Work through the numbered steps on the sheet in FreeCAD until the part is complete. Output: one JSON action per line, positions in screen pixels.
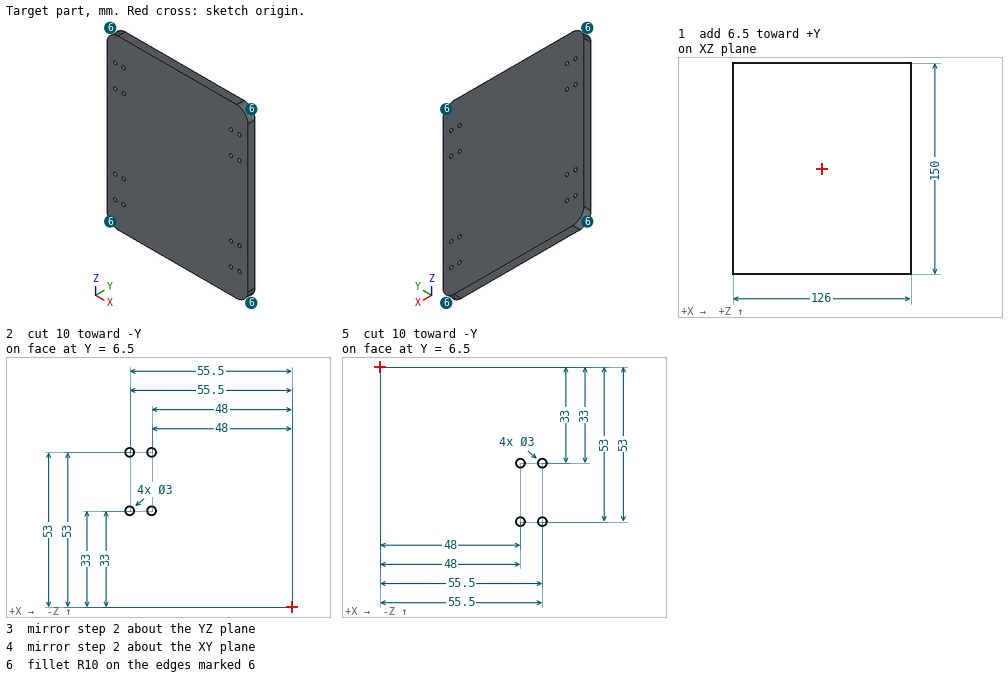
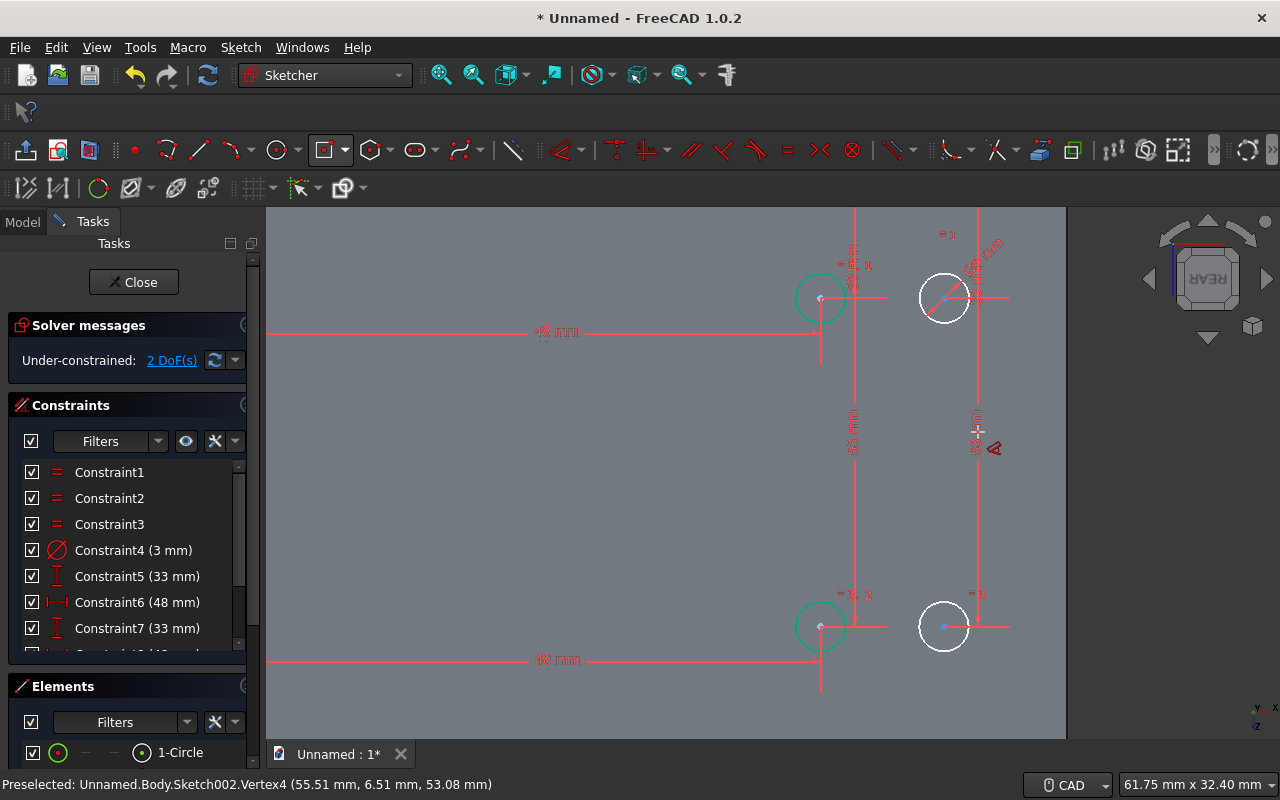
{"action": "left_click", "coordinate": [944, 298]}
{"action": "left_click", "coordinate": [470, 332]}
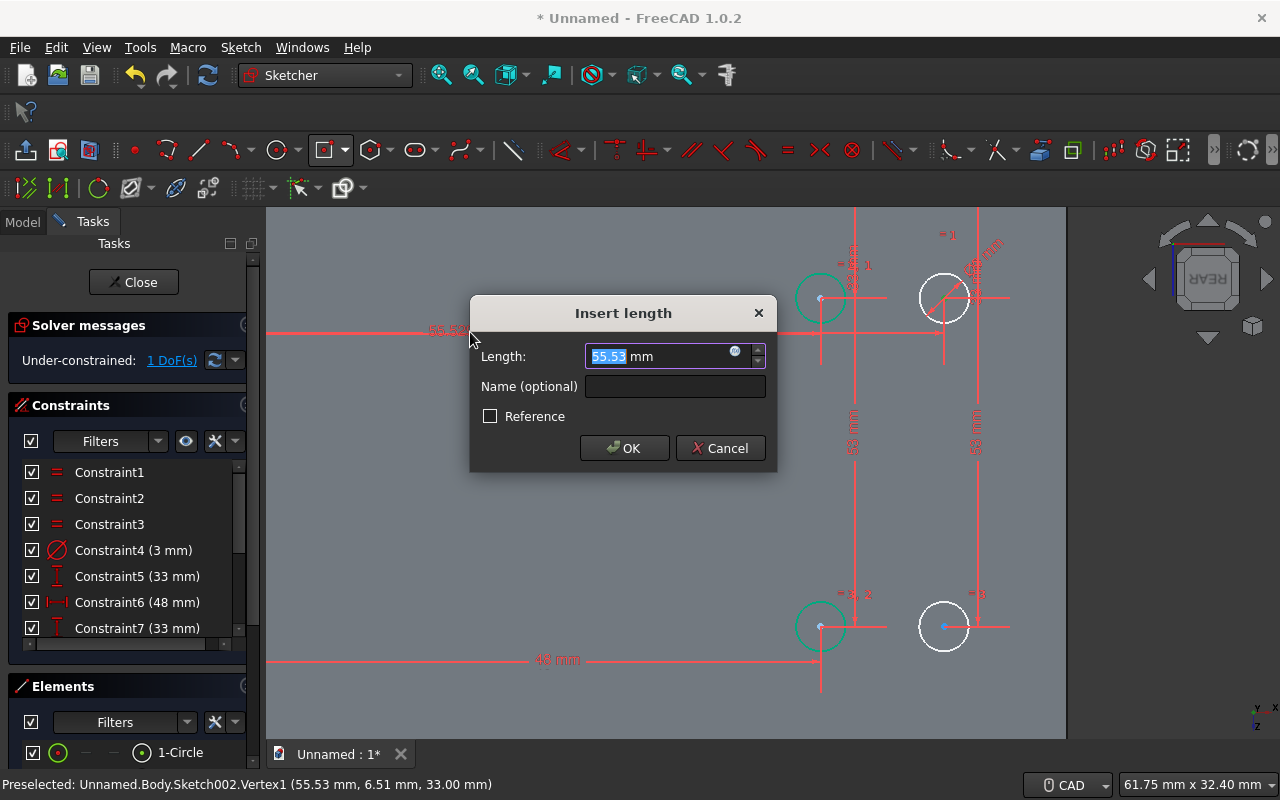
{"action": "type", "text": "55.5"}
{"action": "key", "text": "Return"}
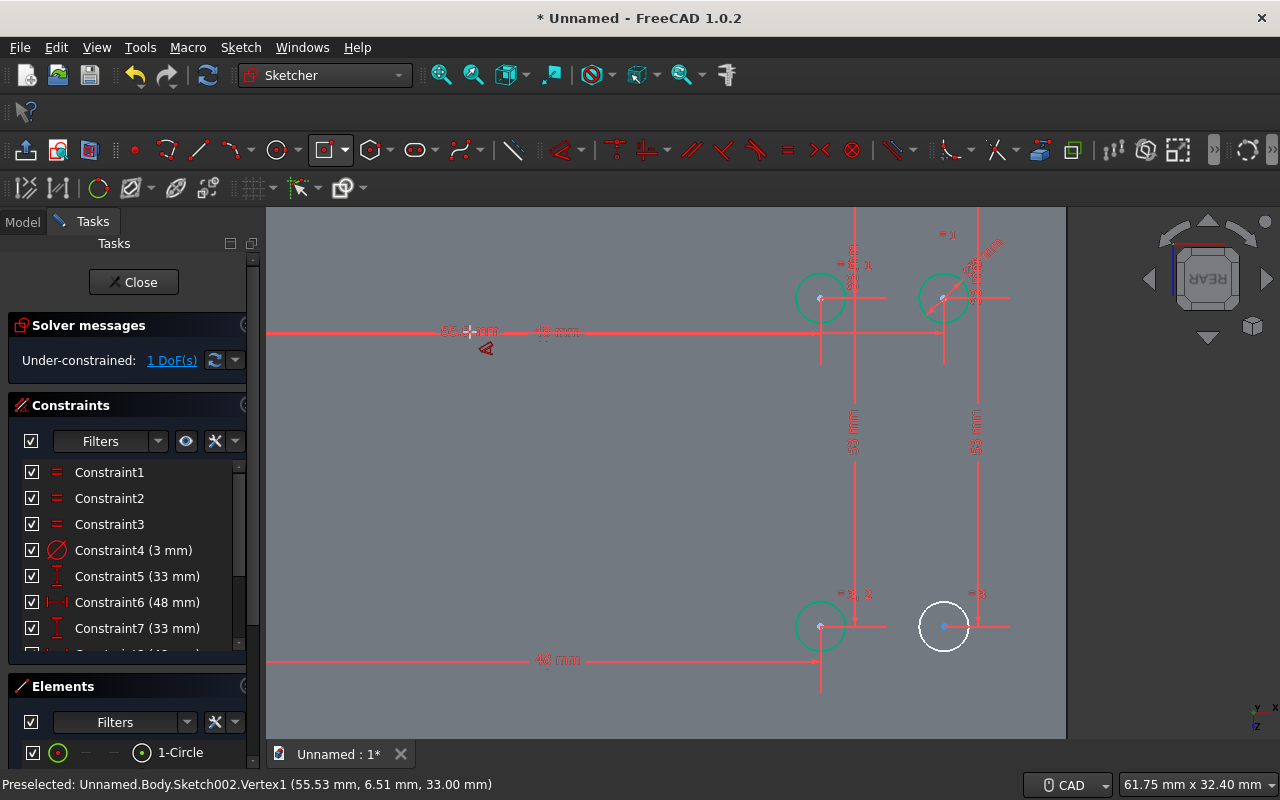
{"action": "left_click", "coordinate": [944, 627]}
{"action": "left_click", "coordinate": [470, 661]}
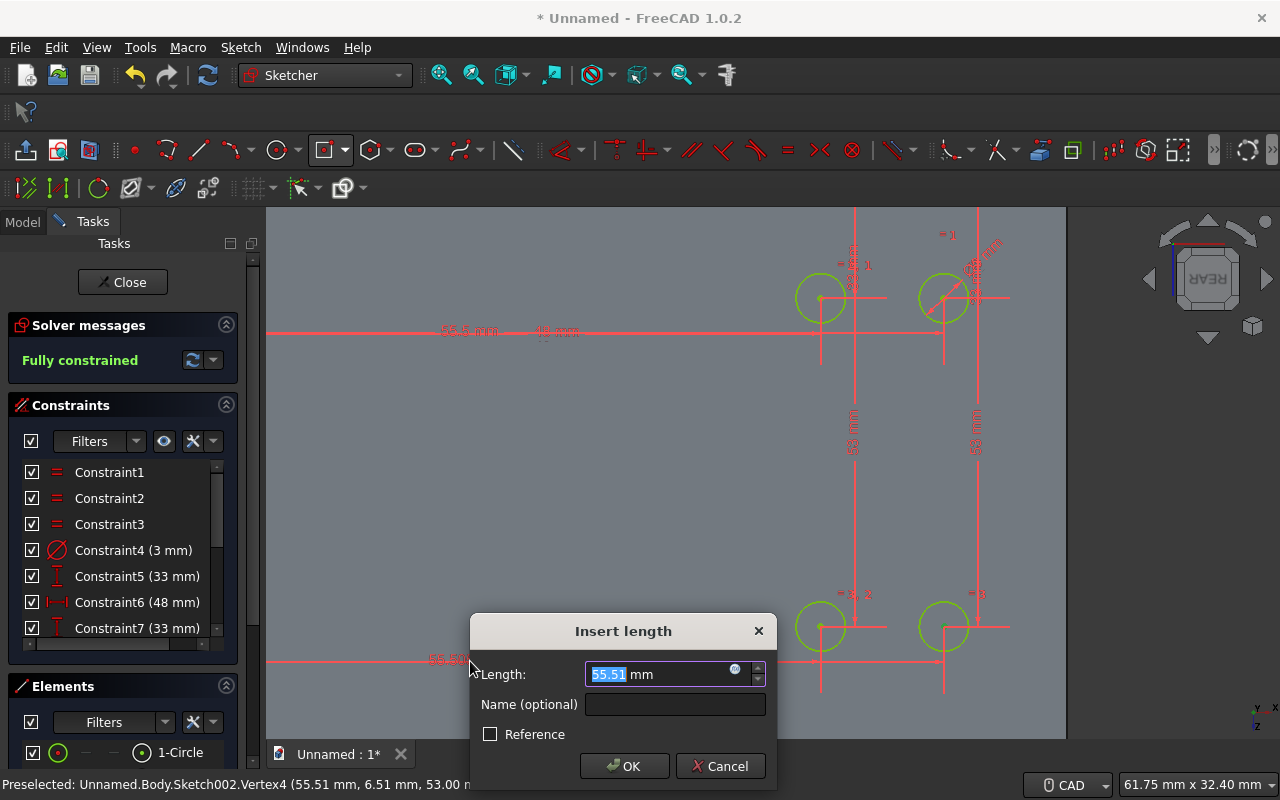
{"action": "type", "text": "55.5"}
{"action": "key", "text": "Return"}
{"action": "key", "text": "Escape"}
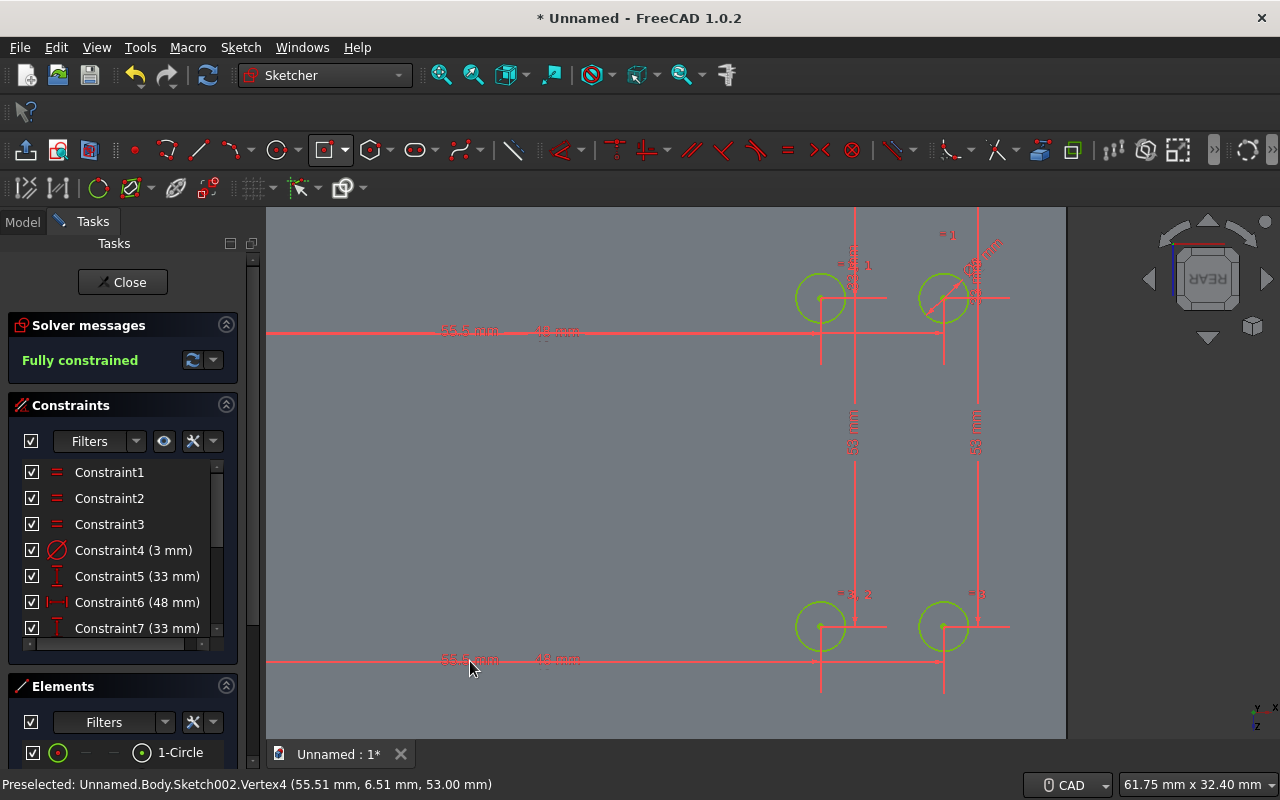
{"action": "left_click", "coordinate": [123, 282]}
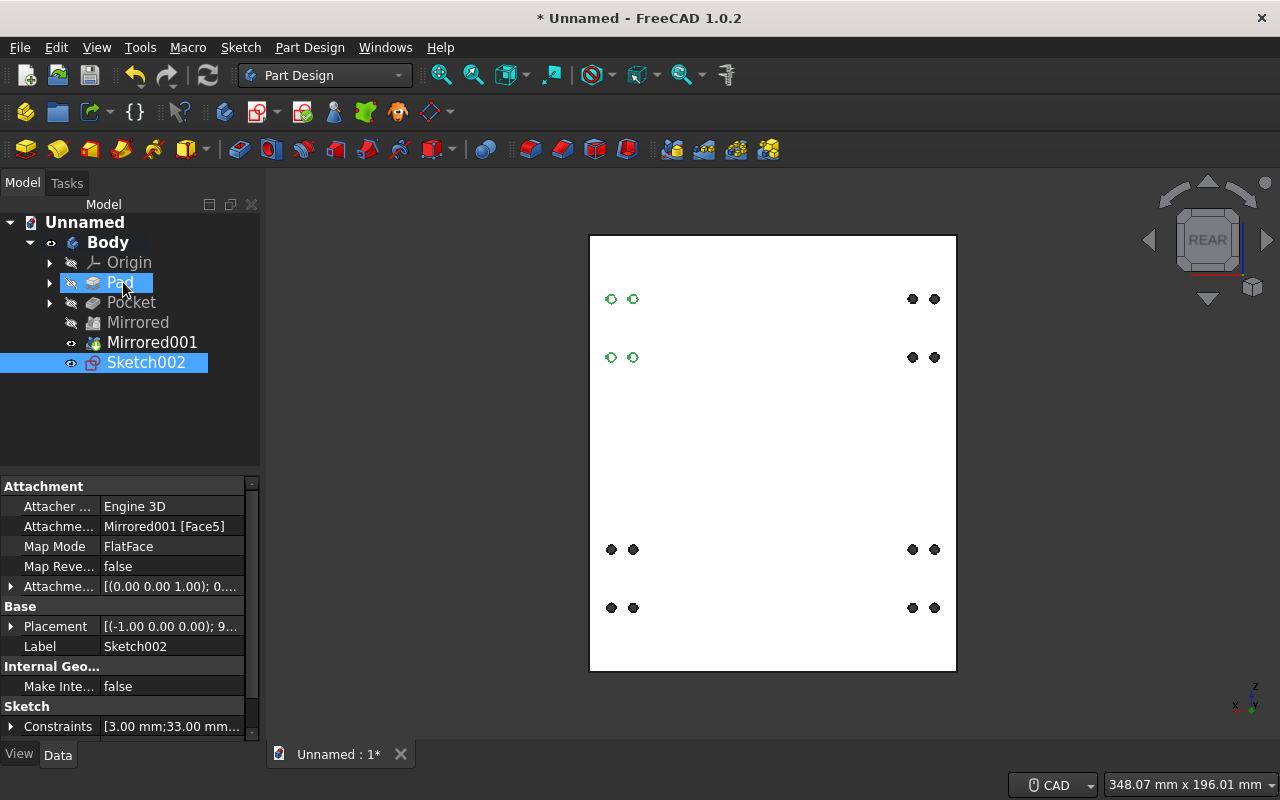
{"action": "left_click", "coordinate": [240, 150]}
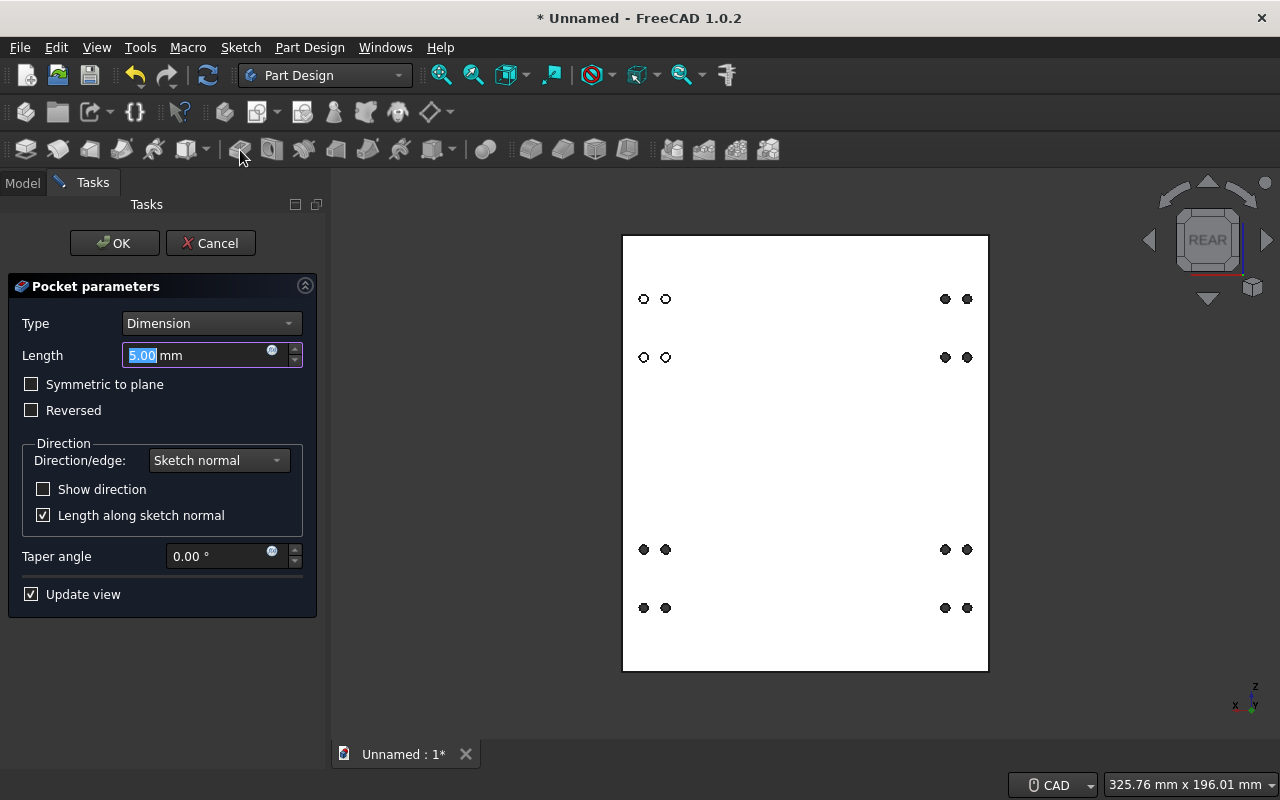
{"action": "type", "text": "10"}
{"action": "key", "text": "Tab"}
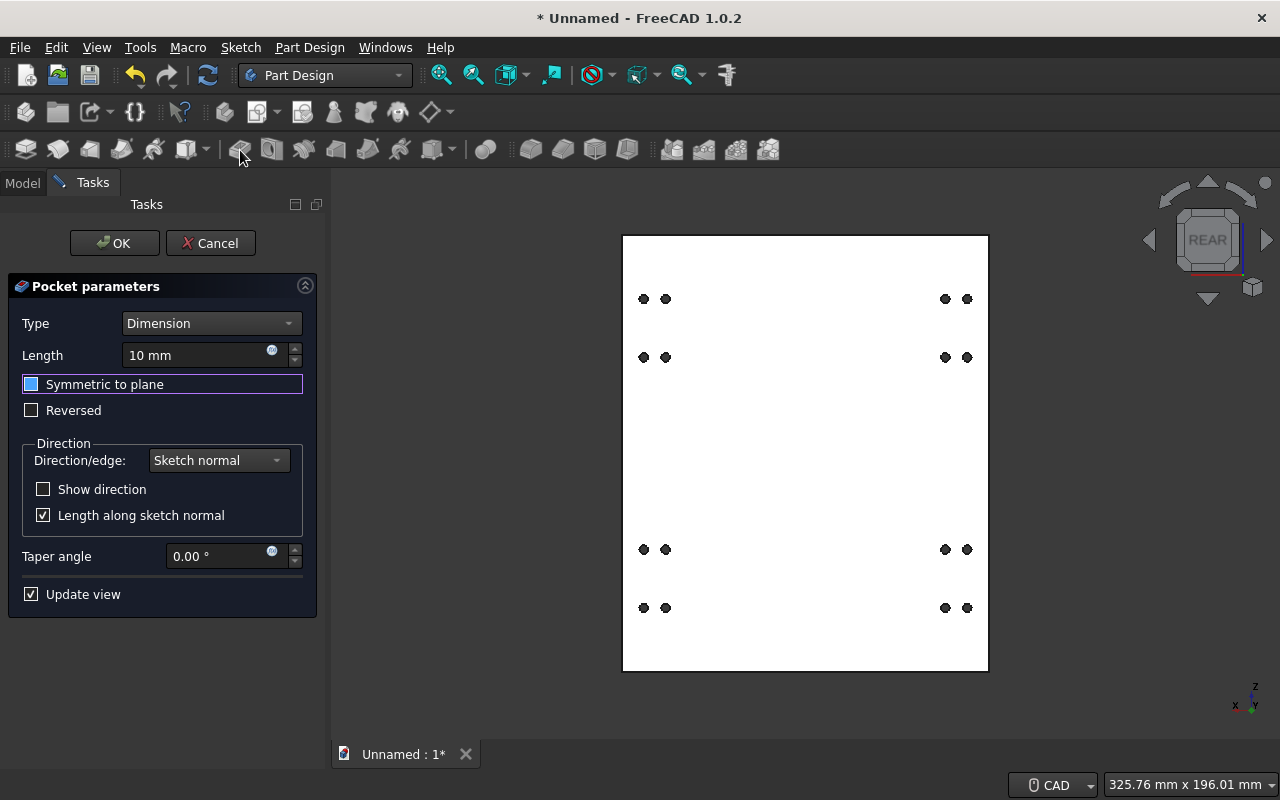
{"action": "left_click", "coordinate": [115, 243]}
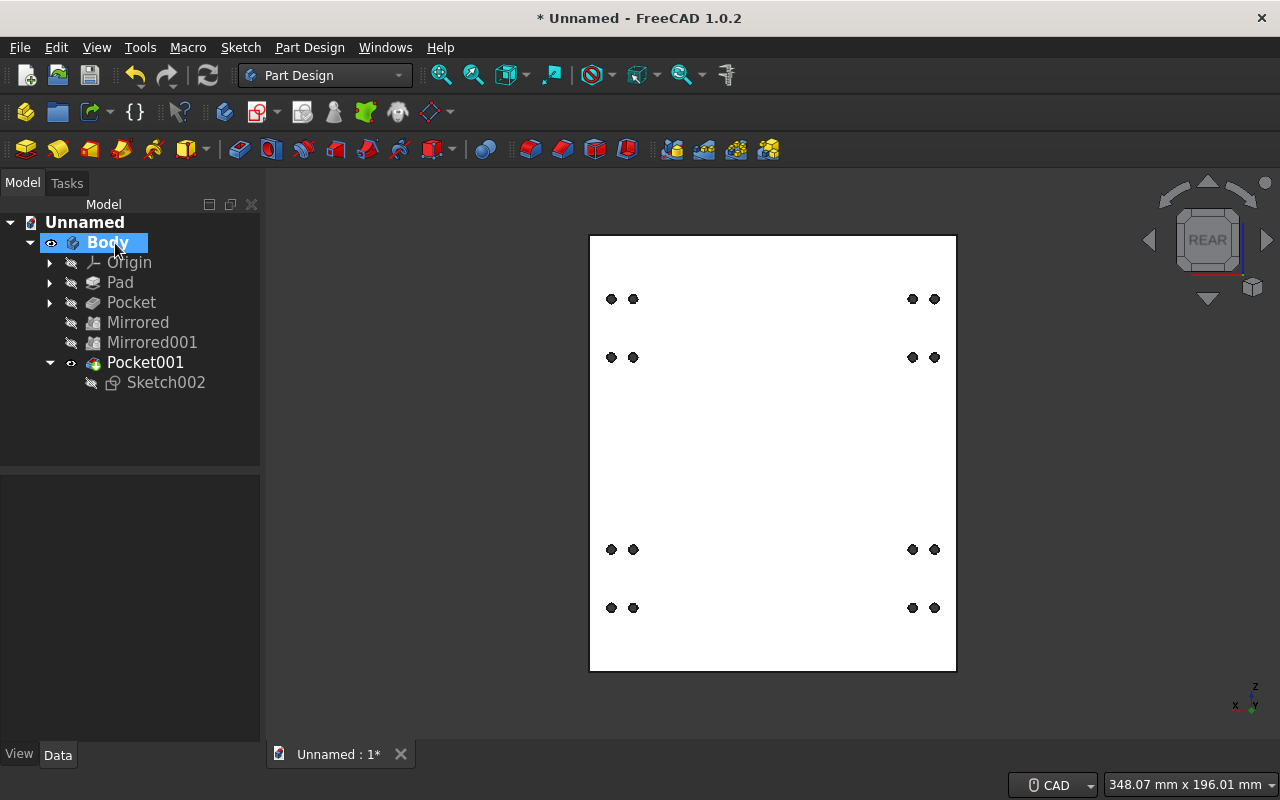
{"action": "scroll", "coordinate": [589, 234], "scroll_direction": "up", "scroll_amount": 4}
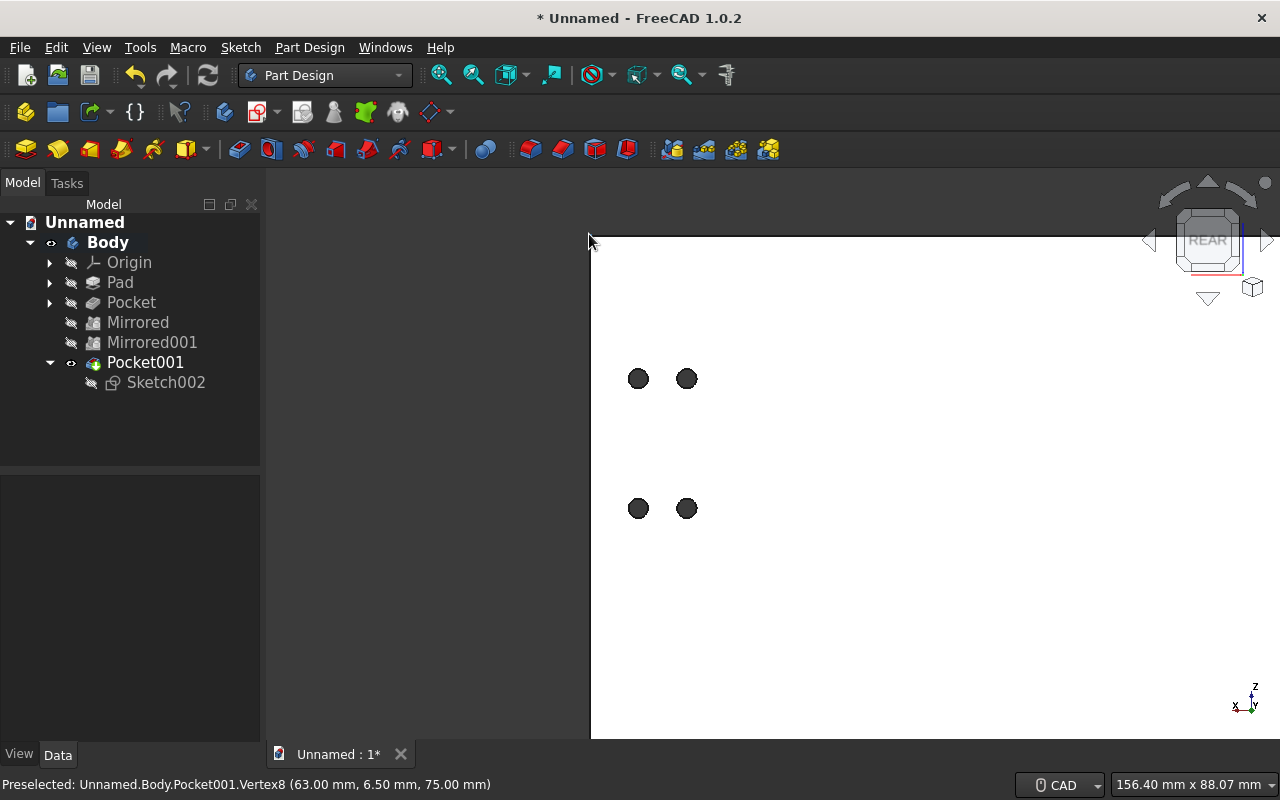
{"action": "left_click", "coordinate": [442, 76]}